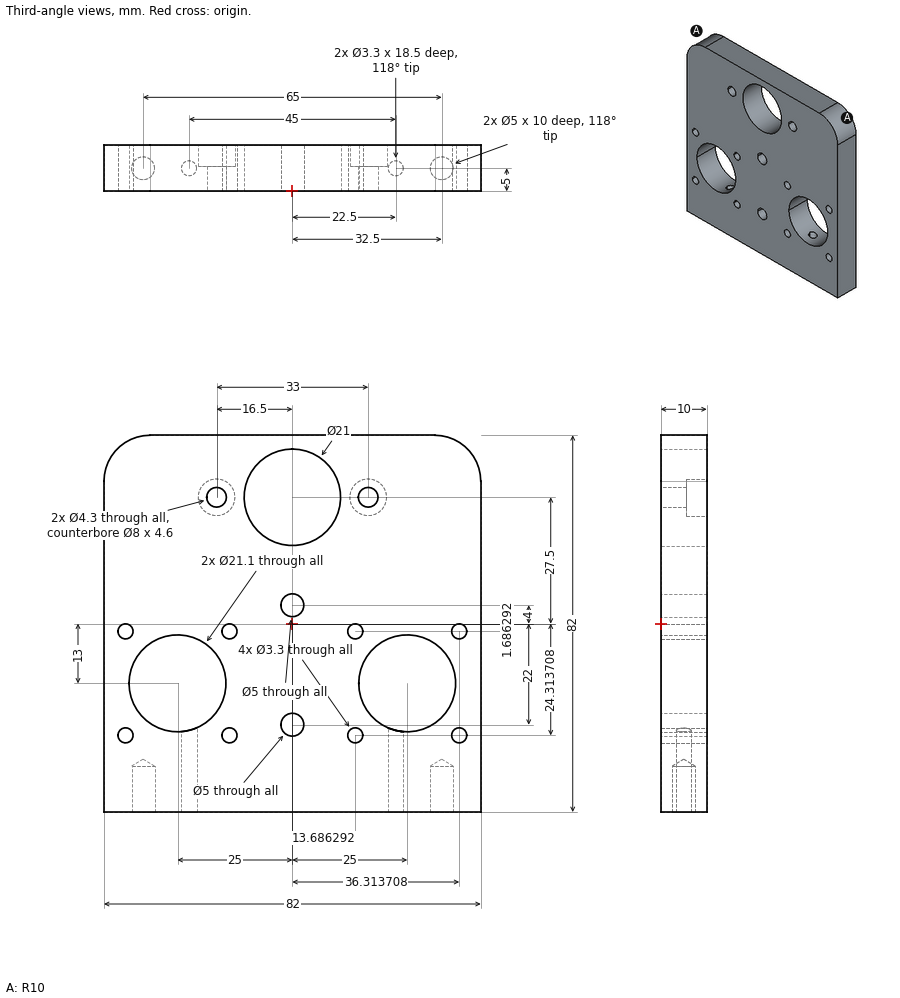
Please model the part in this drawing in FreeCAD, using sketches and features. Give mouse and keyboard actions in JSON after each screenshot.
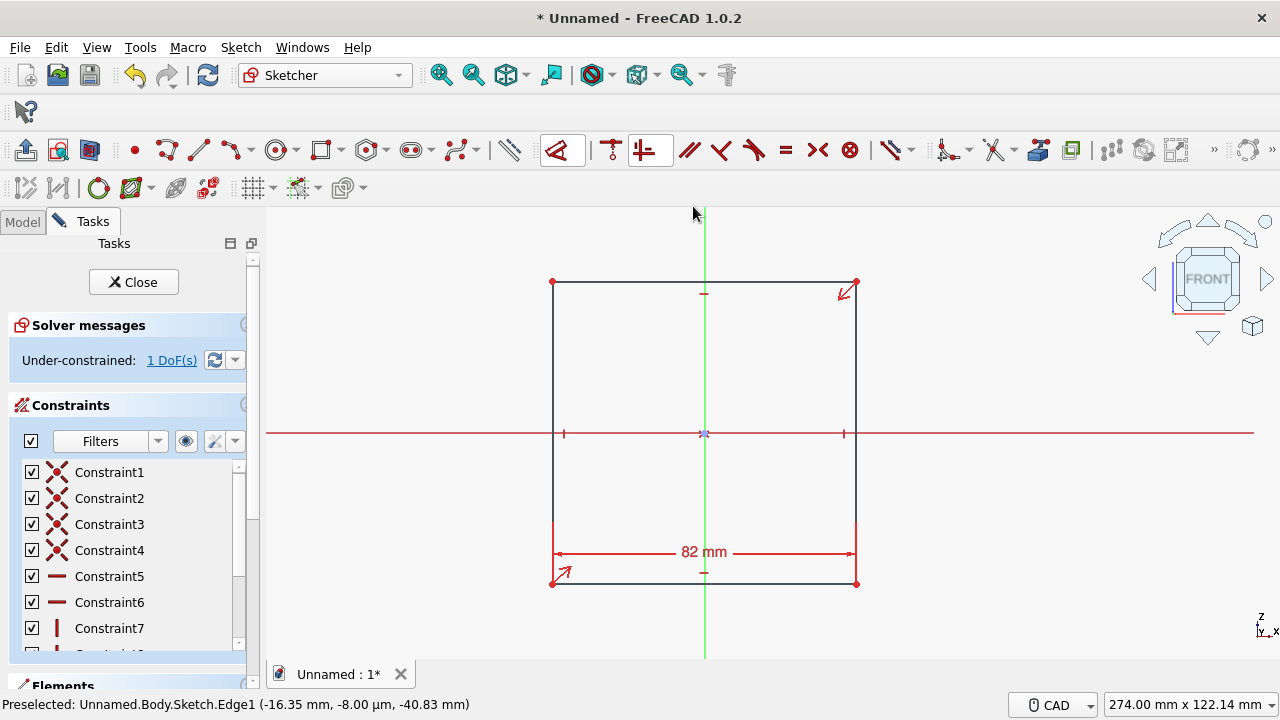
{"action": "left_click", "coordinate": [856, 494]}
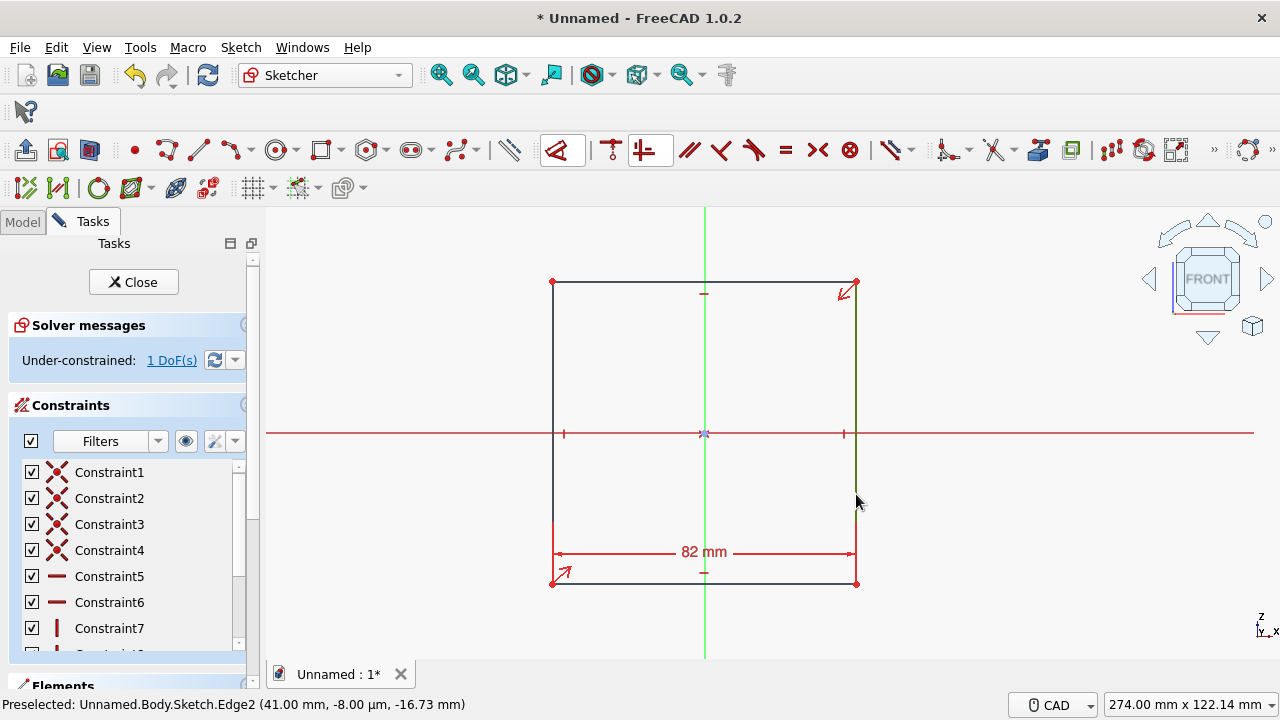
{"action": "left_click", "coordinate": [580, 150]}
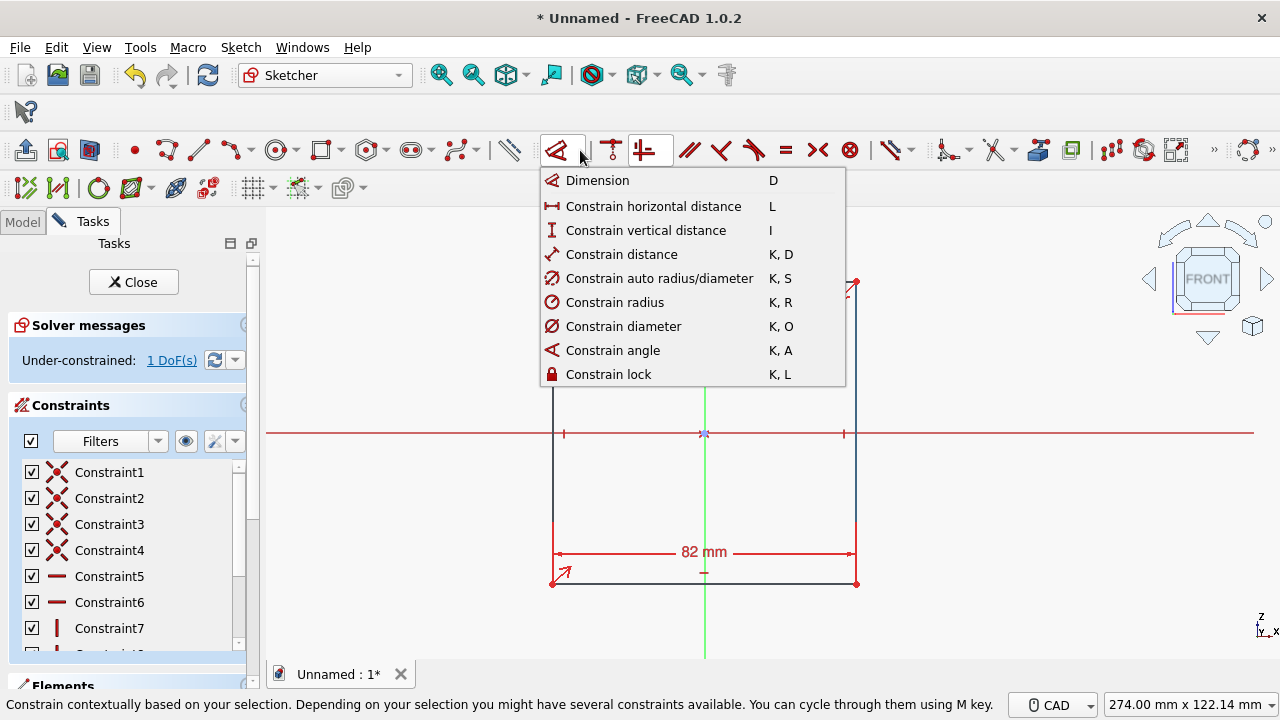
{"action": "left_click", "coordinate": [693, 230]}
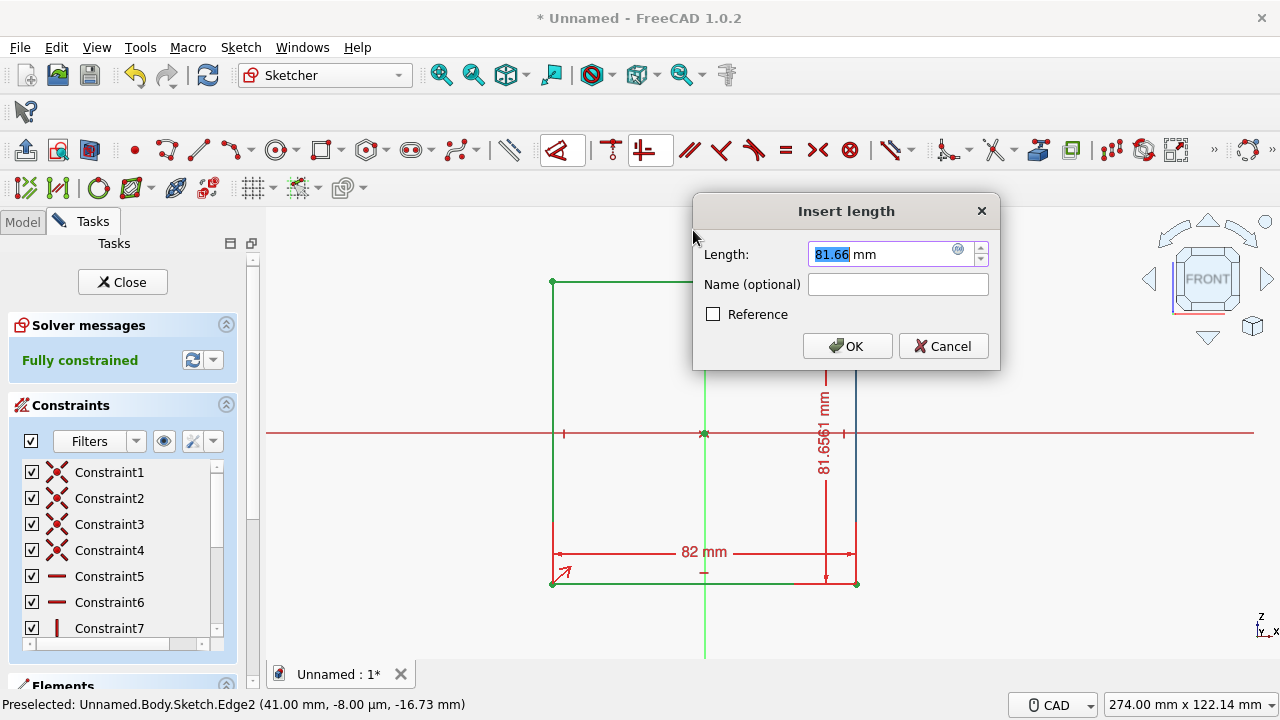
{"action": "type", "text": "82"}
{"action": "key", "text": "Return"}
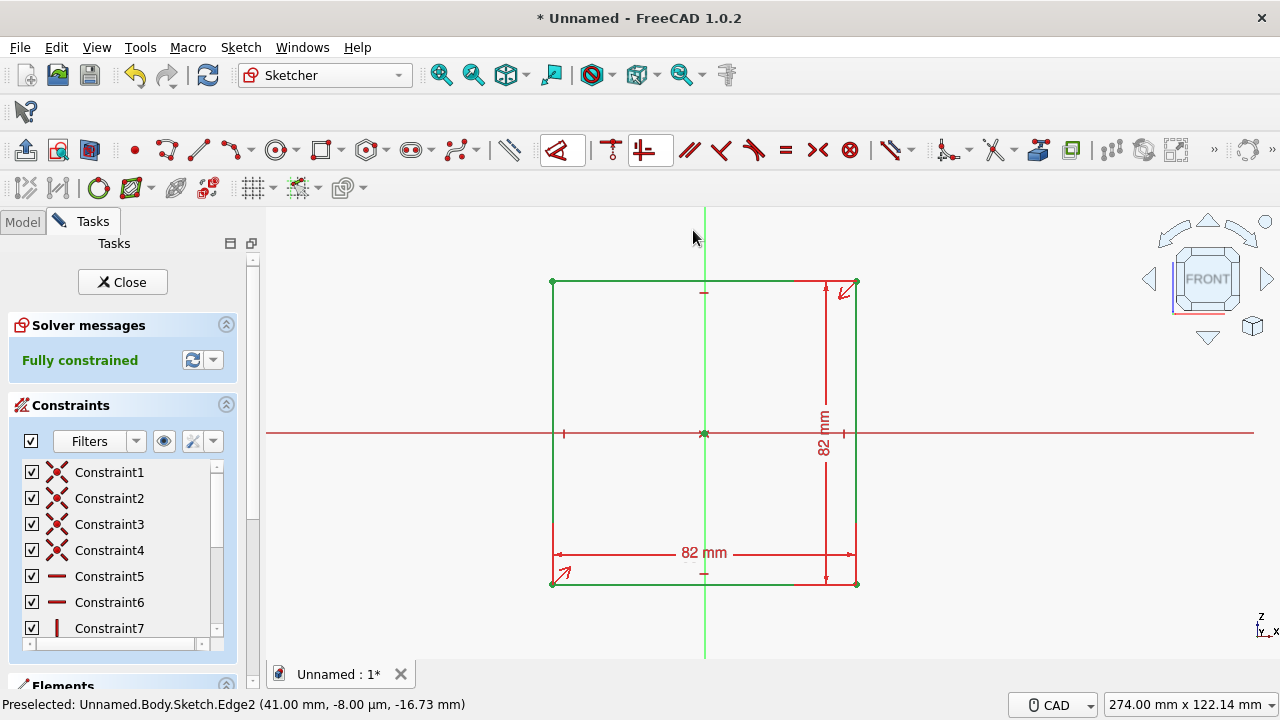
{"action": "left_click", "coordinate": [123, 282]}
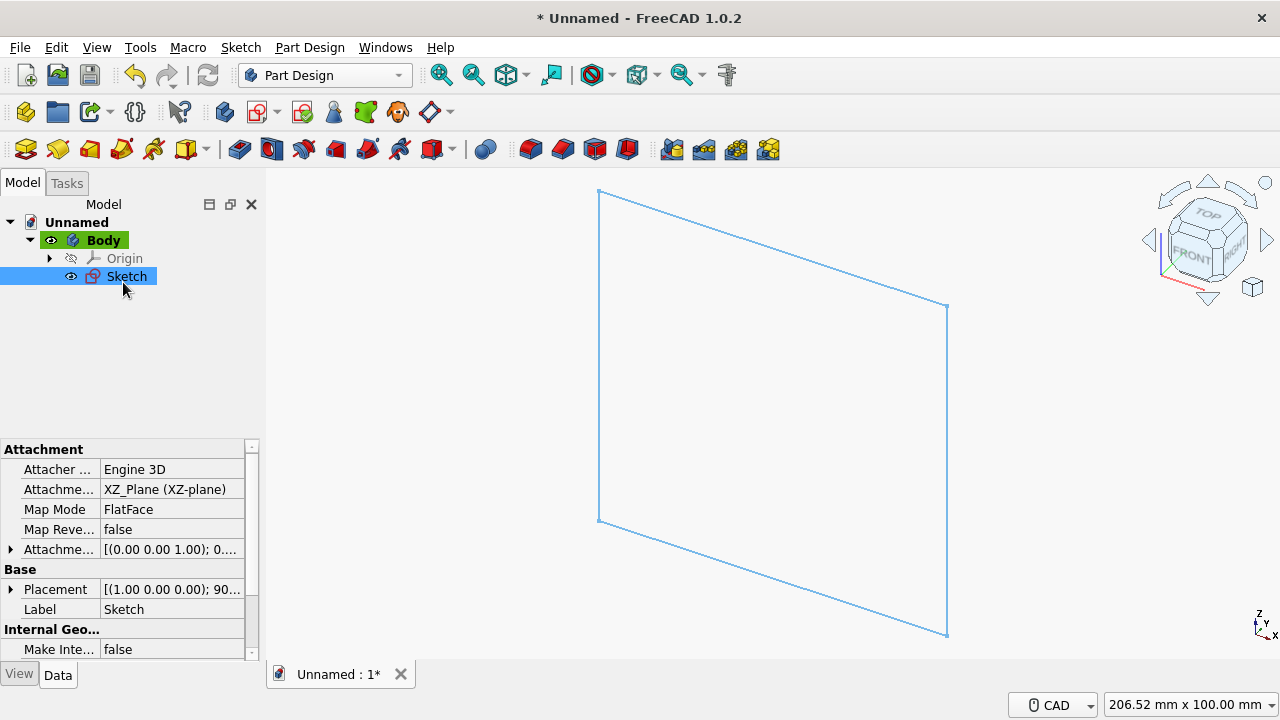
{"action": "left_click", "coordinate": [26, 150]}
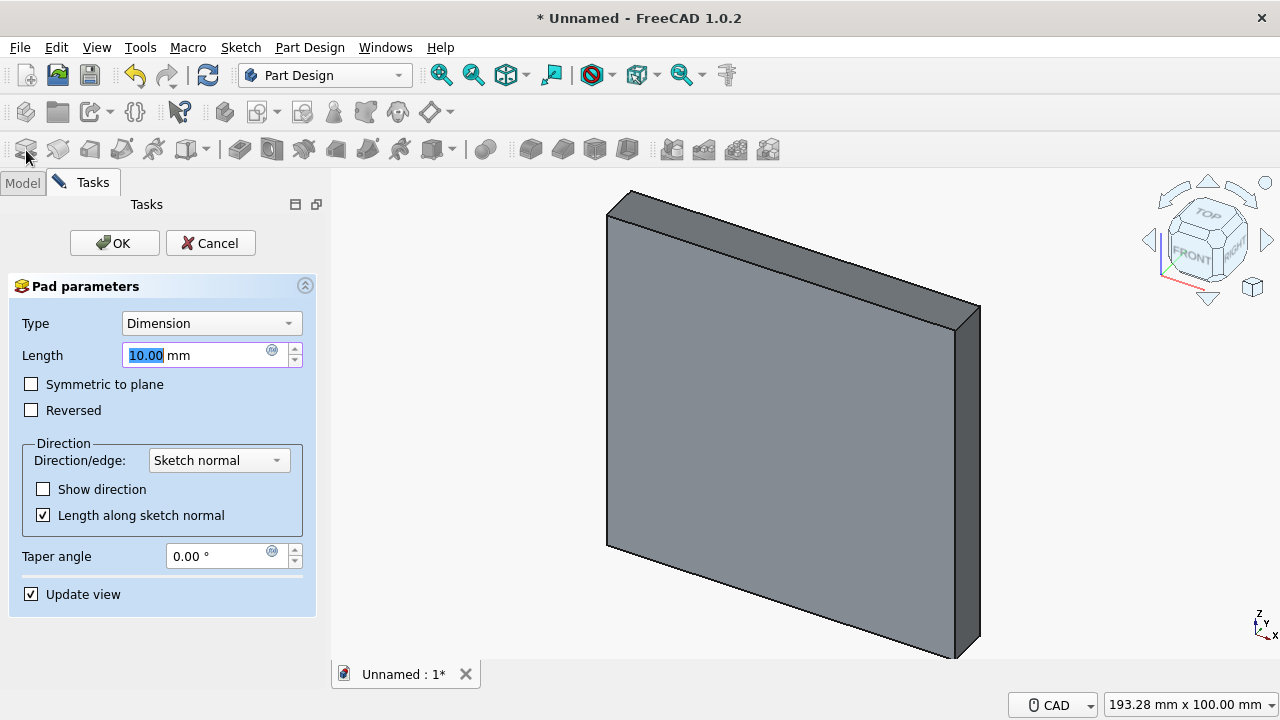
{"action": "type", "text": "10"}
{"action": "key", "text": "Tab"}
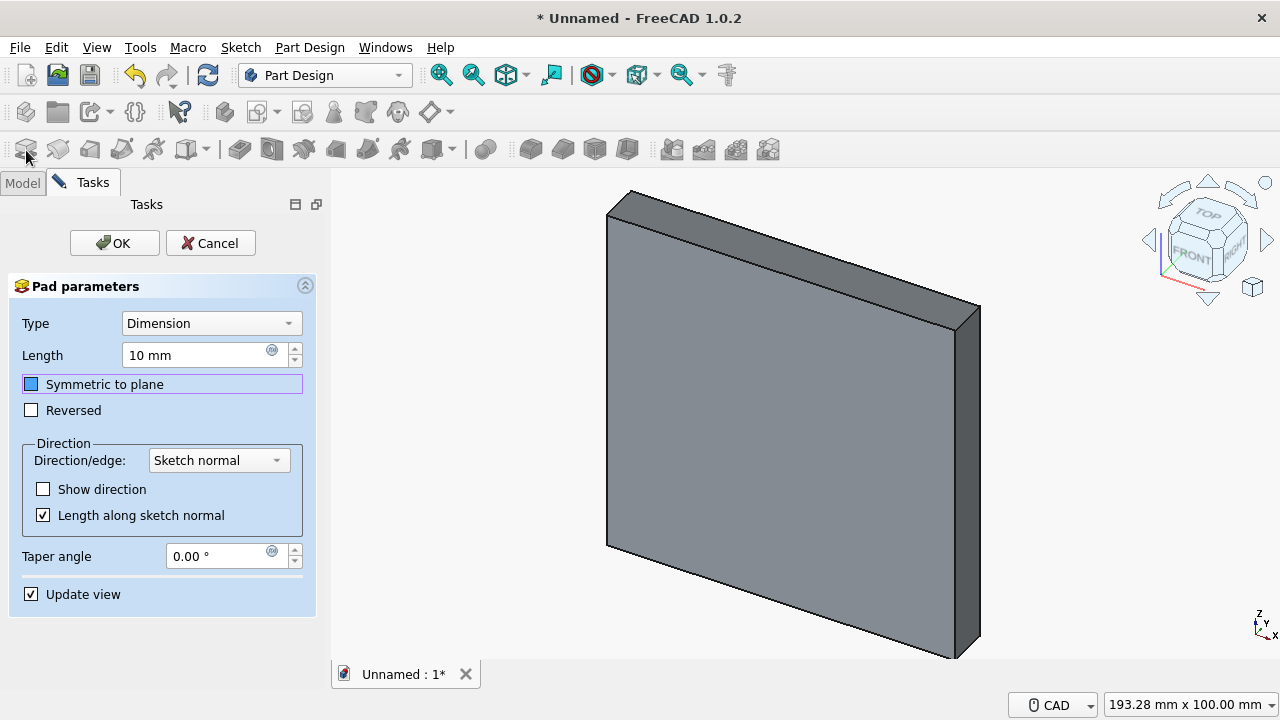
{"action": "left_click", "coordinate": [30, 410]}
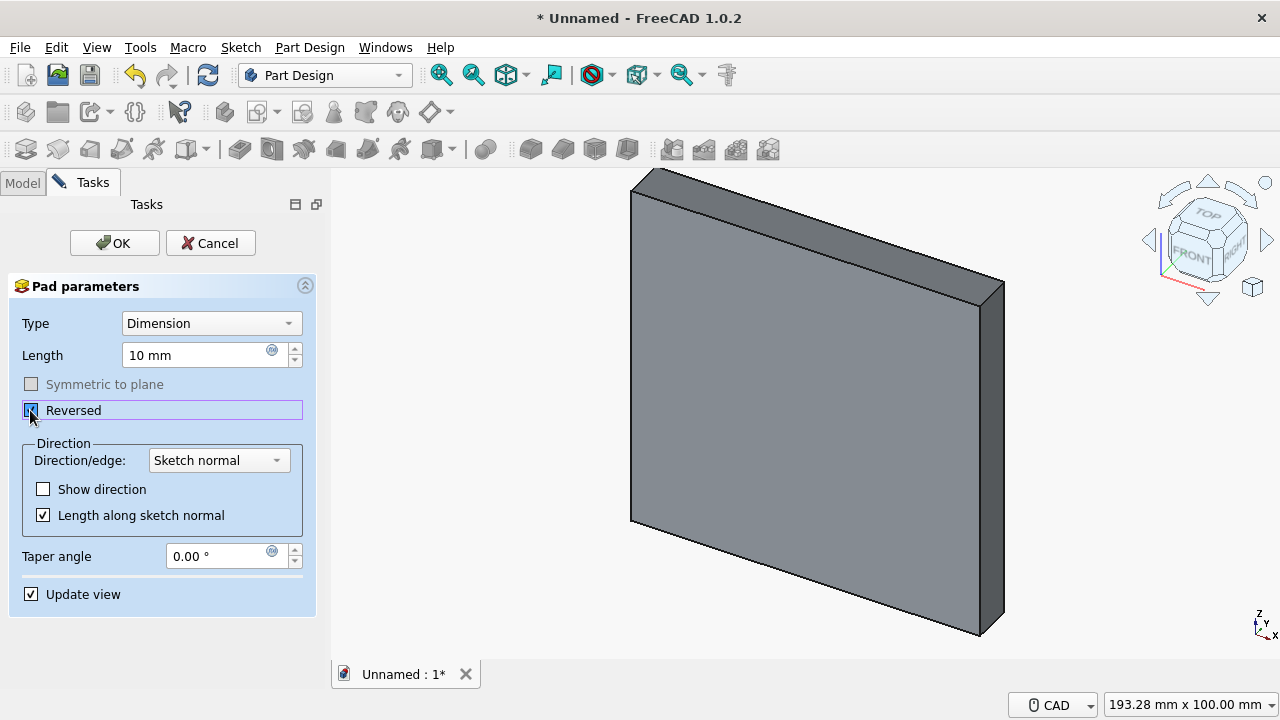
{"action": "left_click", "coordinate": [115, 243]}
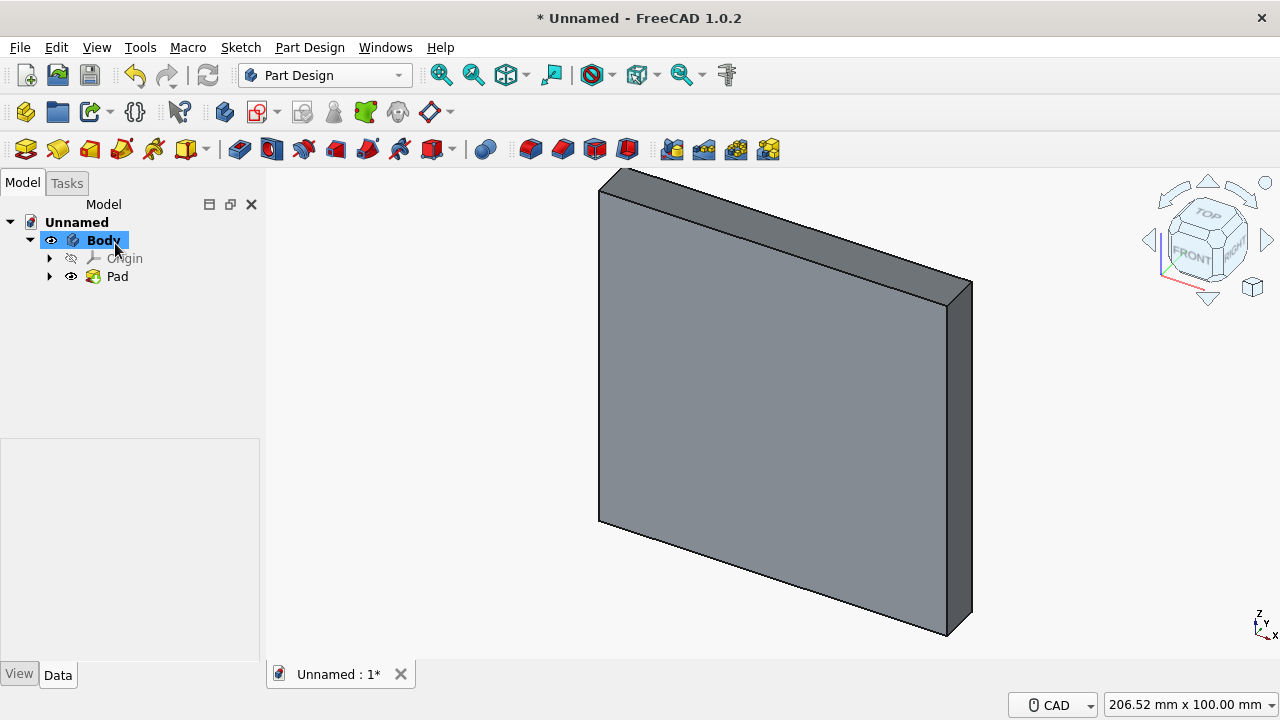
{"action": "left_click", "coordinate": [442, 76]}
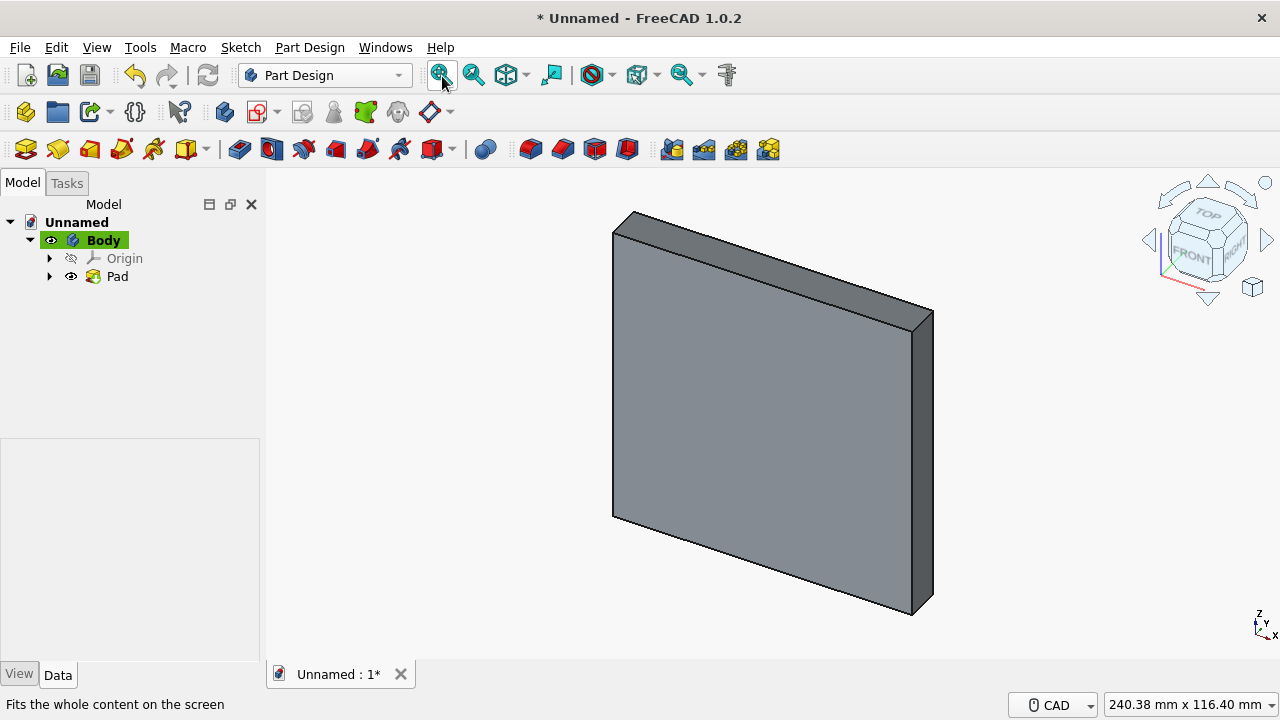
{"action": "key", "text": "4"}